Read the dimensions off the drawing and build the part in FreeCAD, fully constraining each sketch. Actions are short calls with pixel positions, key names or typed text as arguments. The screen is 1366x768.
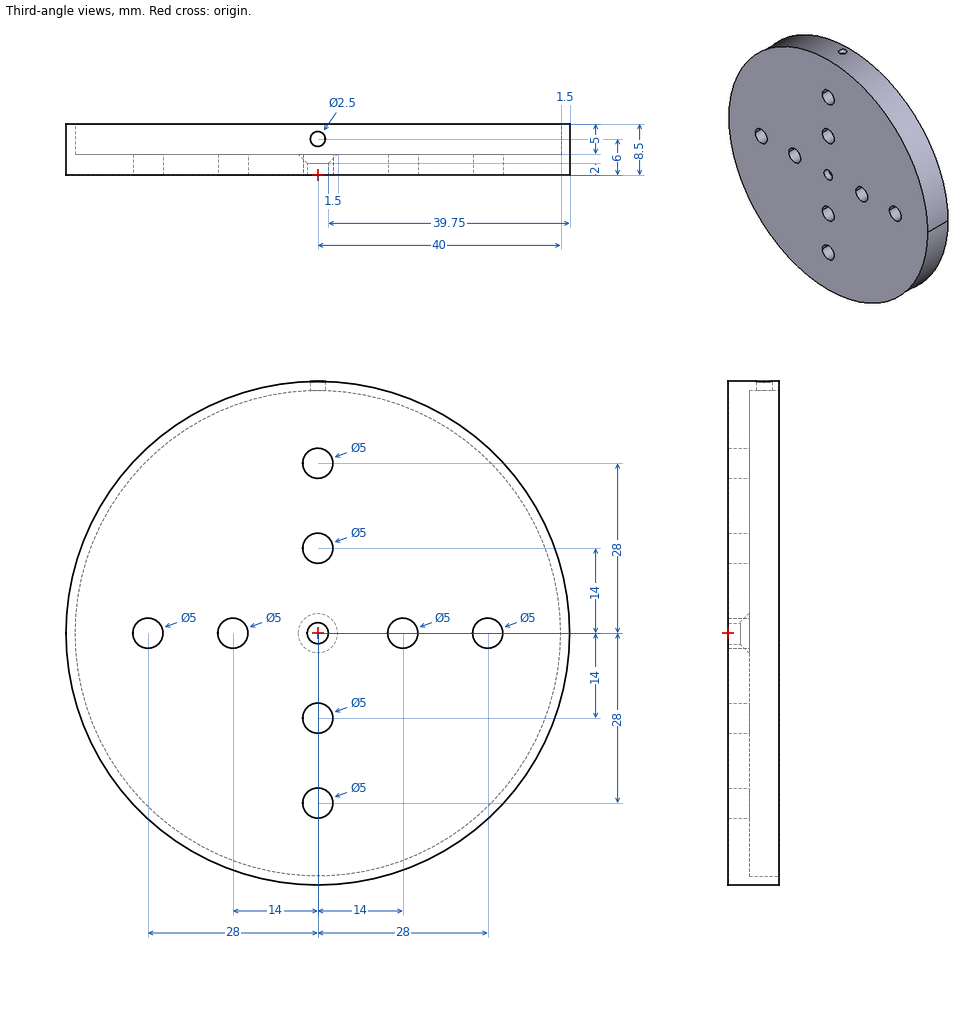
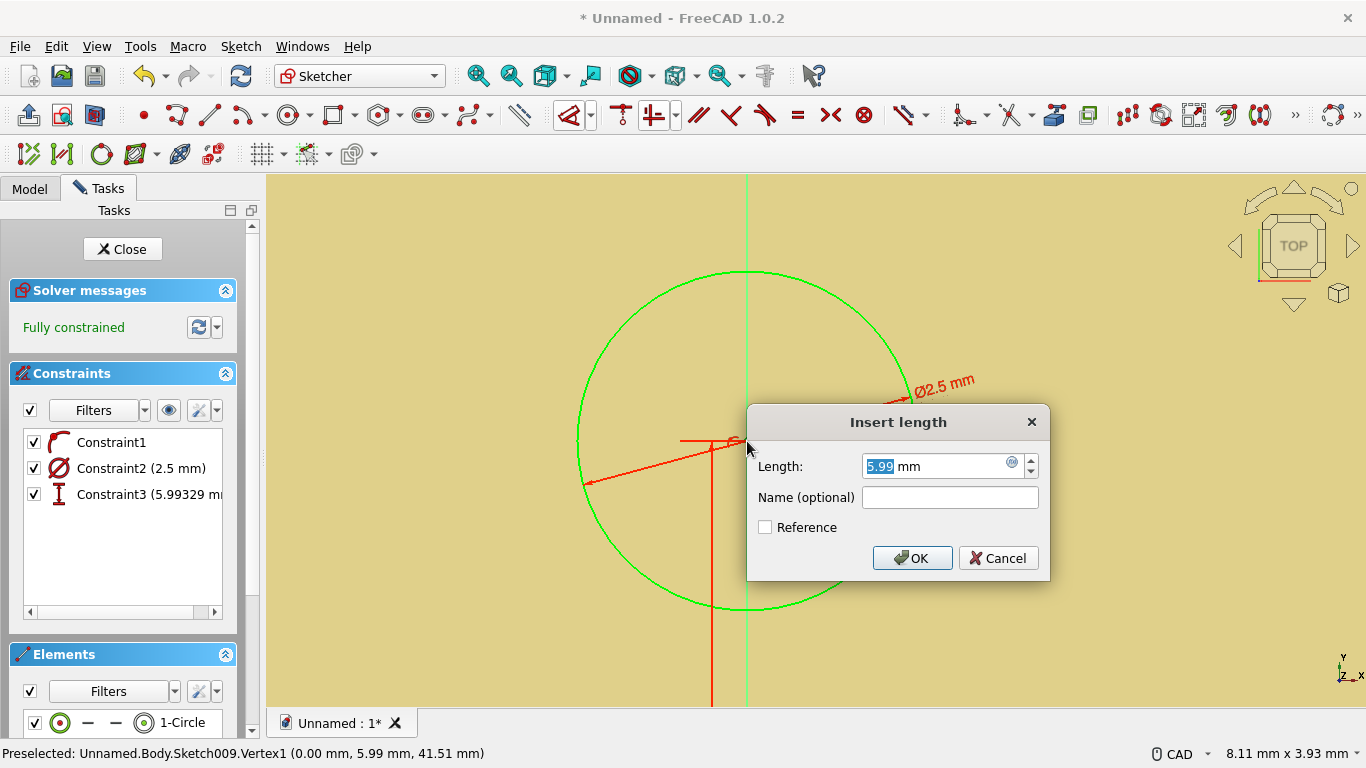
text(6)
key(Return)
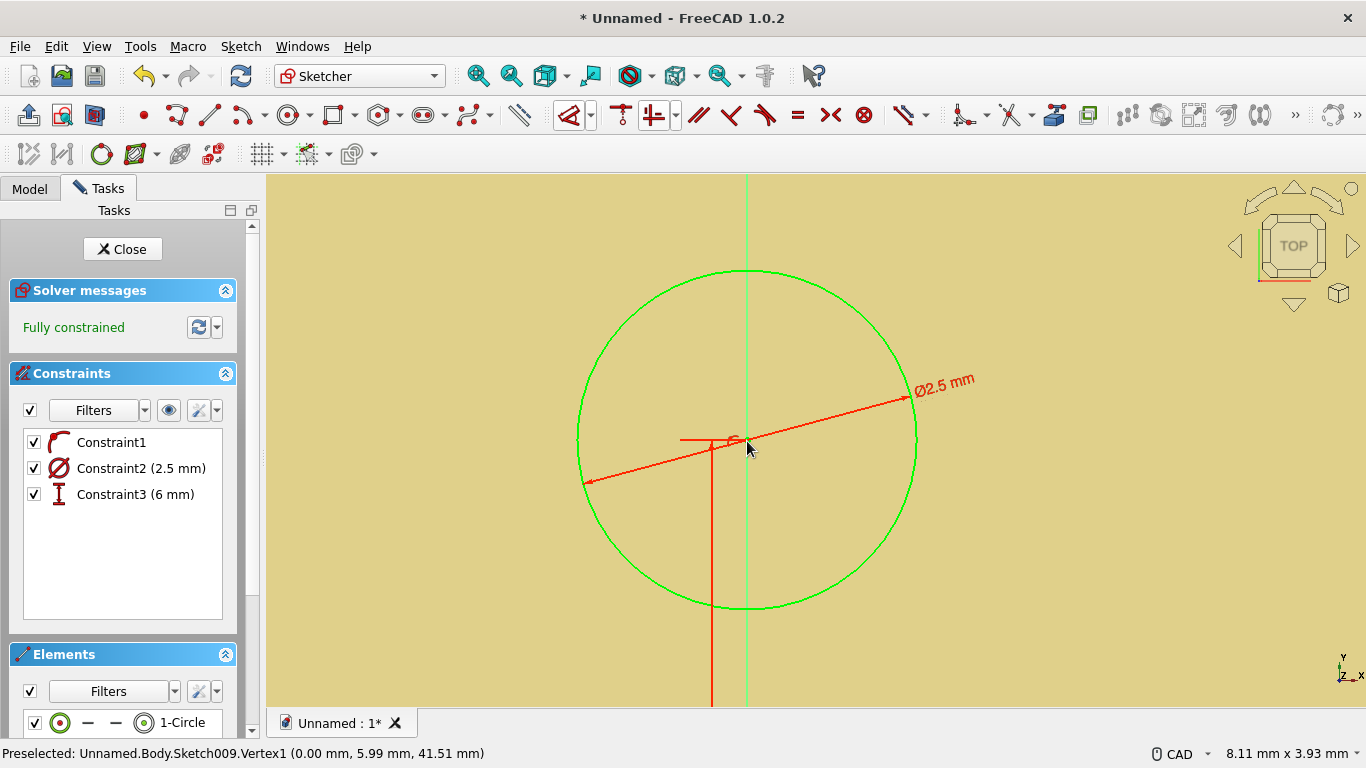
click(123, 249)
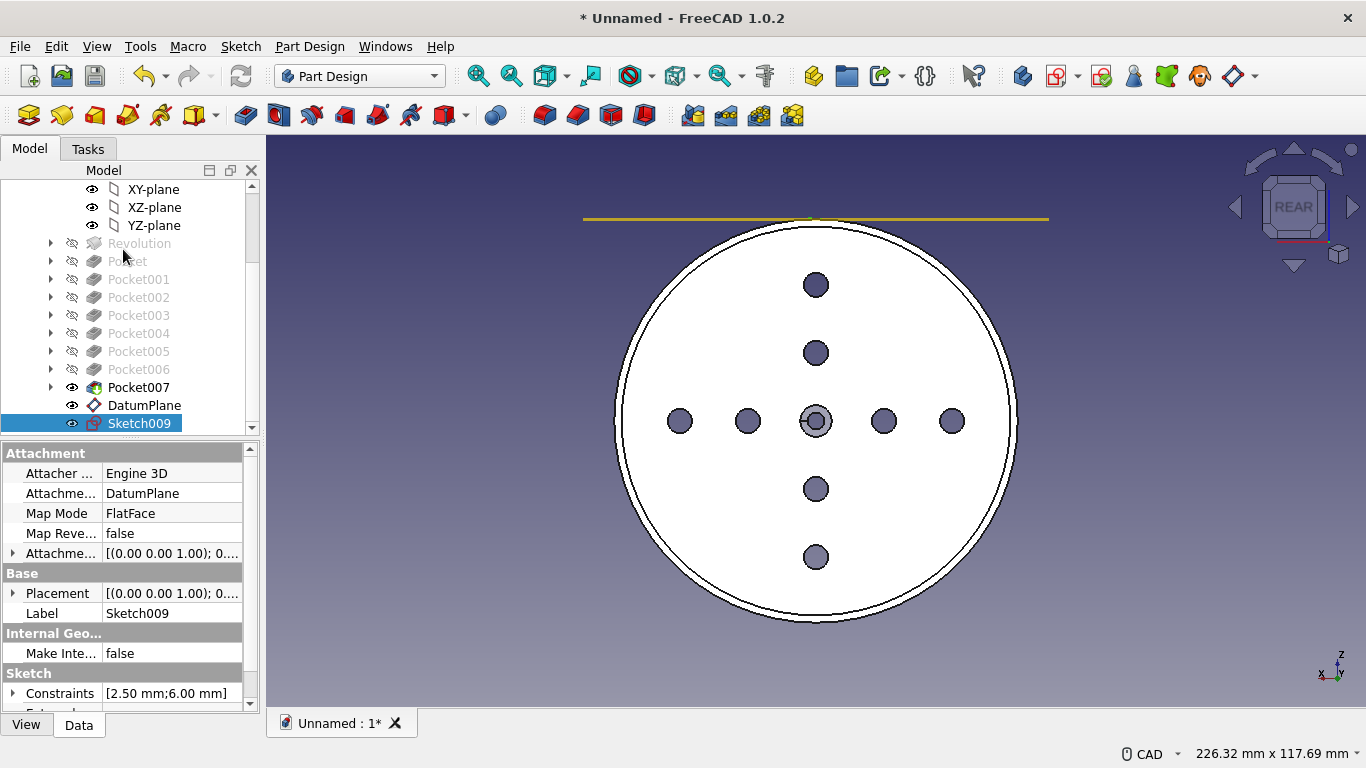
click(246, 116)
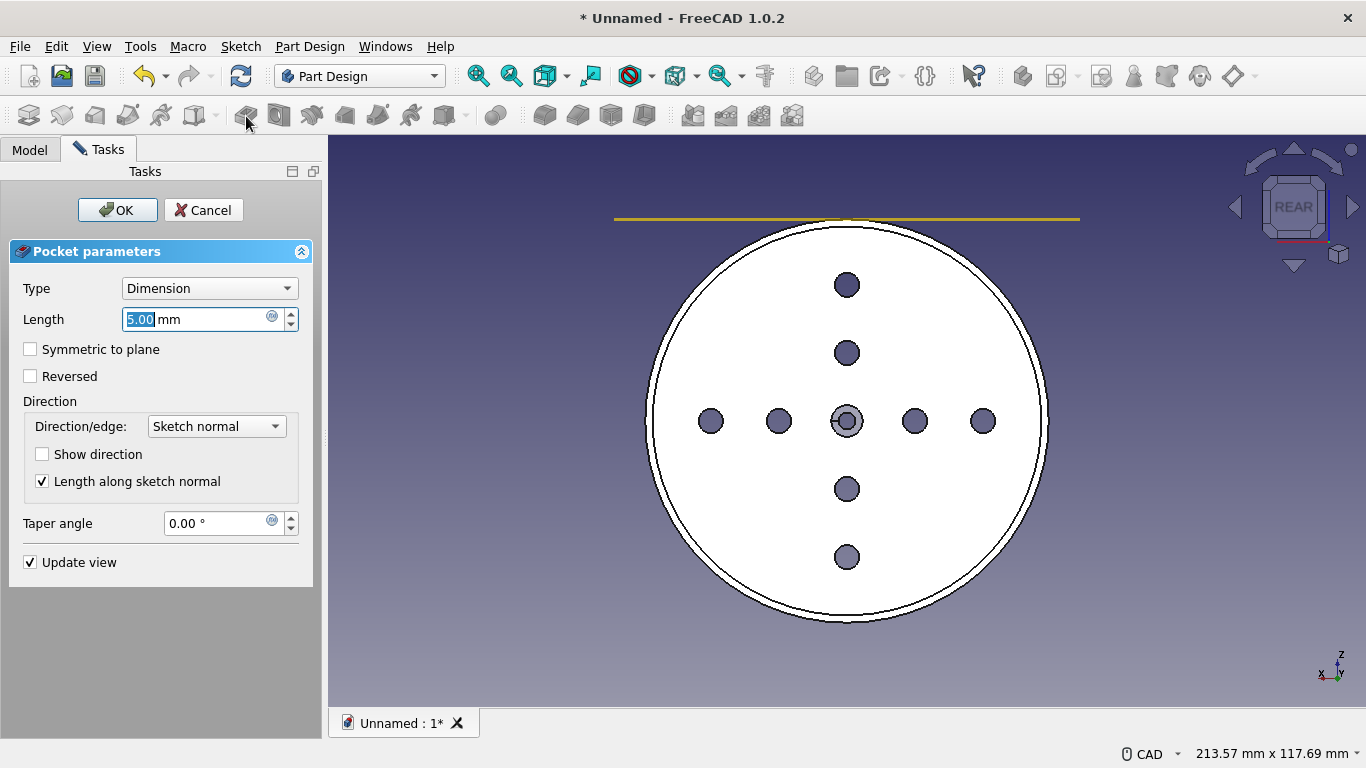
click(210, 288)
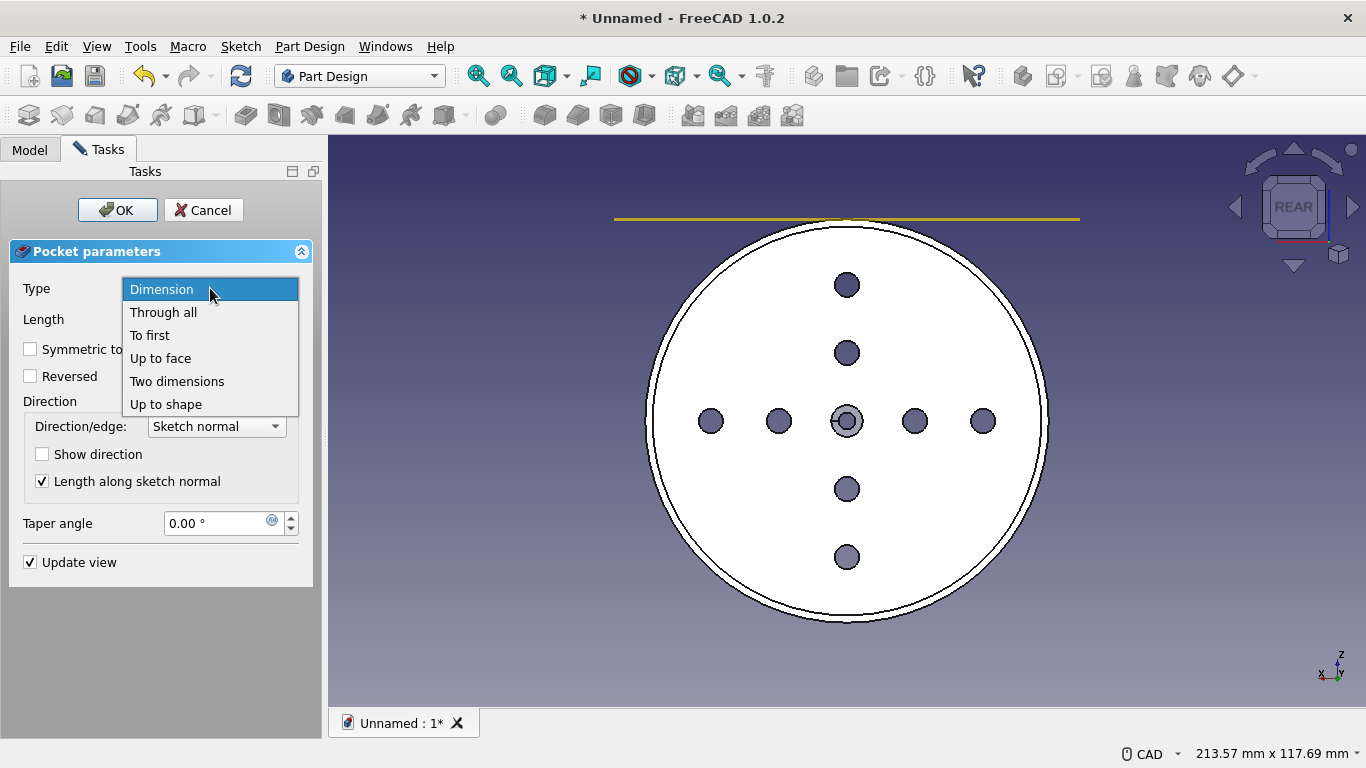
click(208, 336)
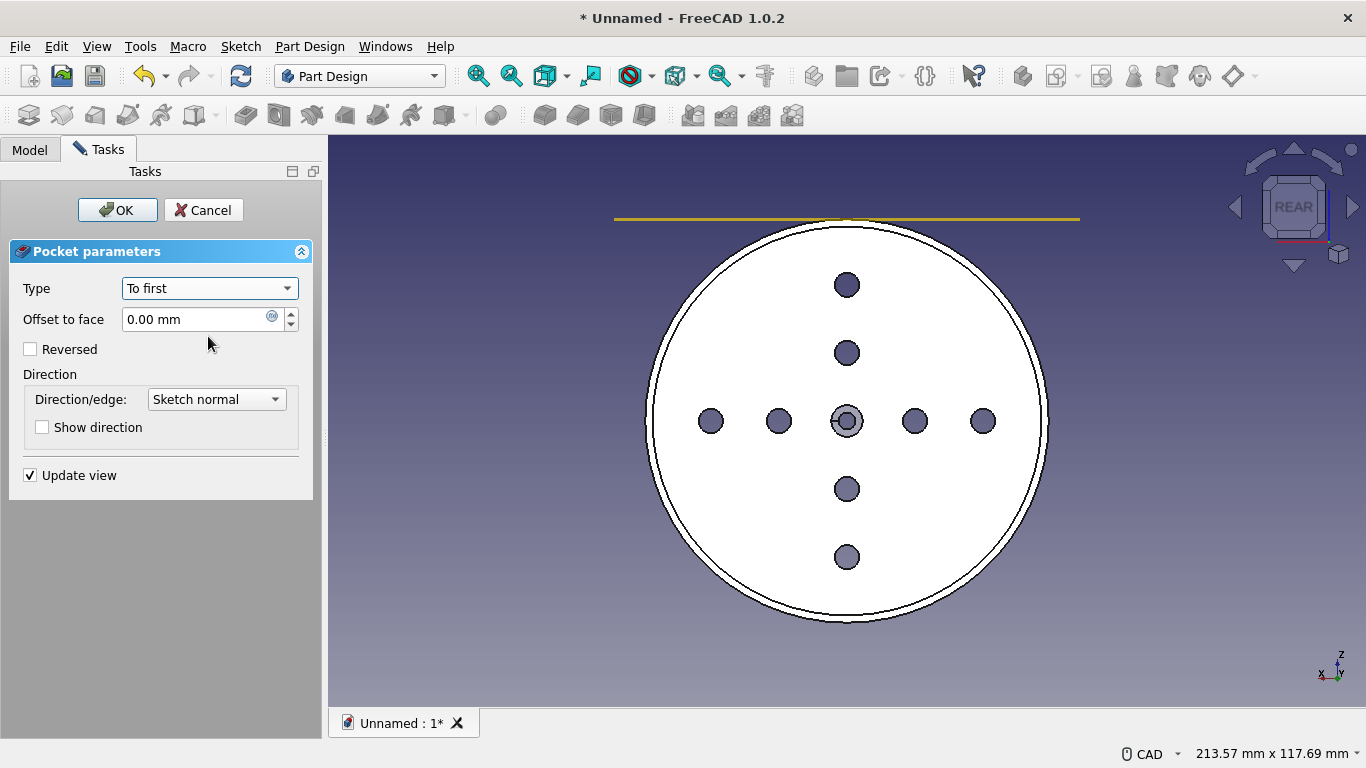
click(118, 210)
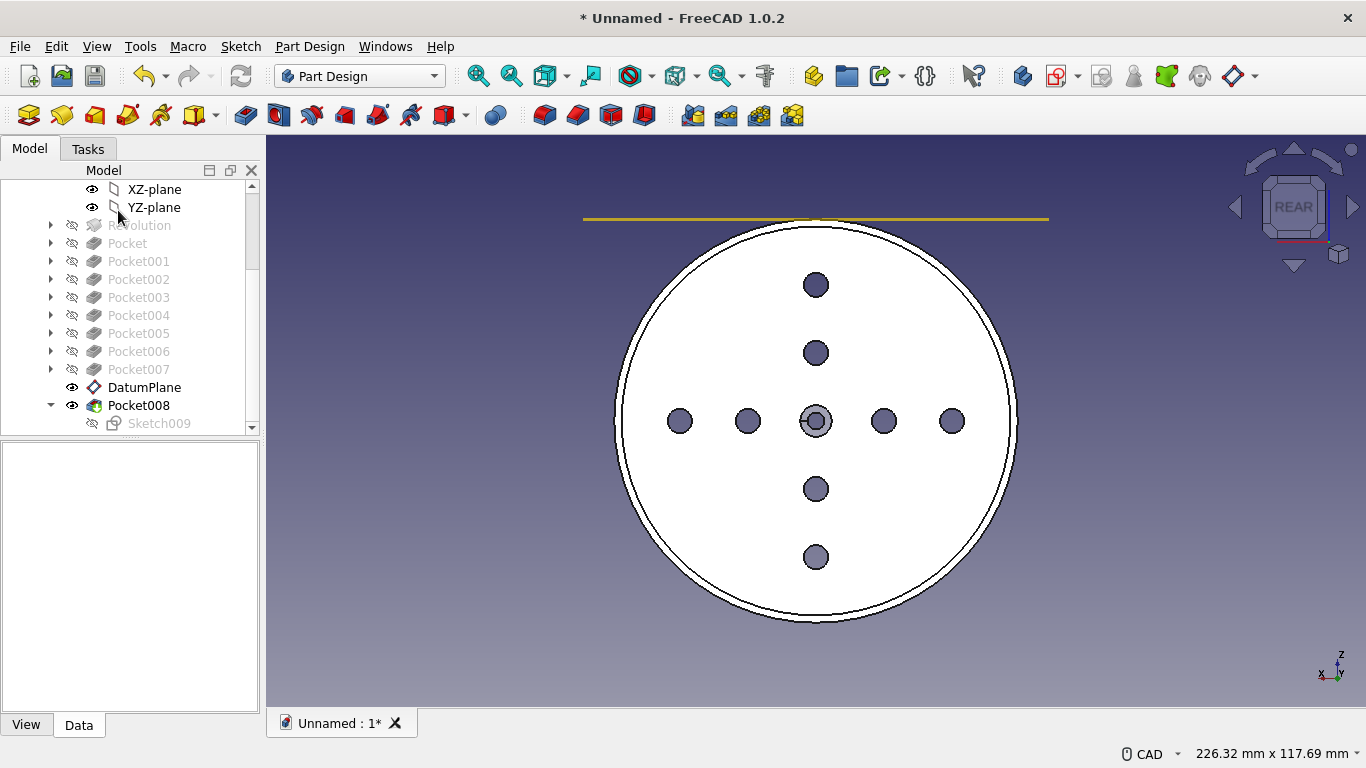
click(117, 387)
key(space)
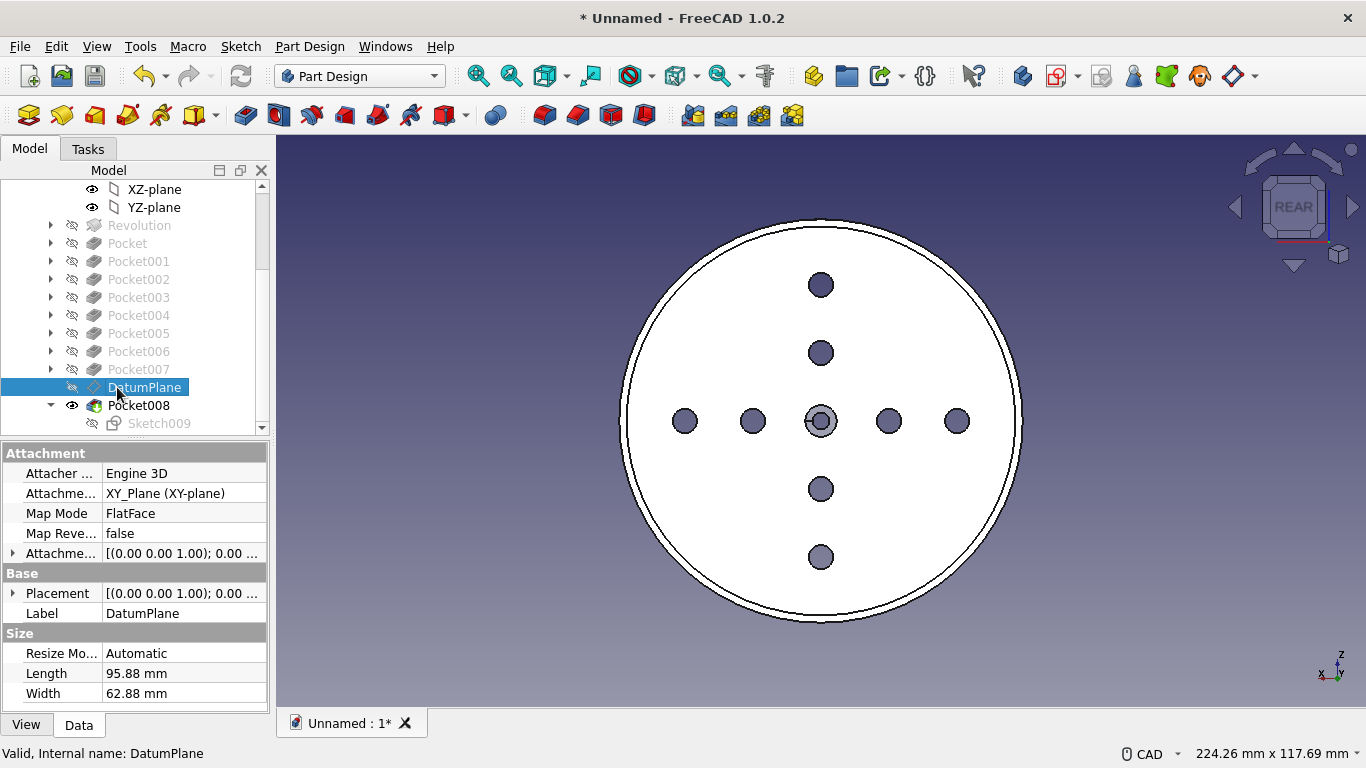
key(0)